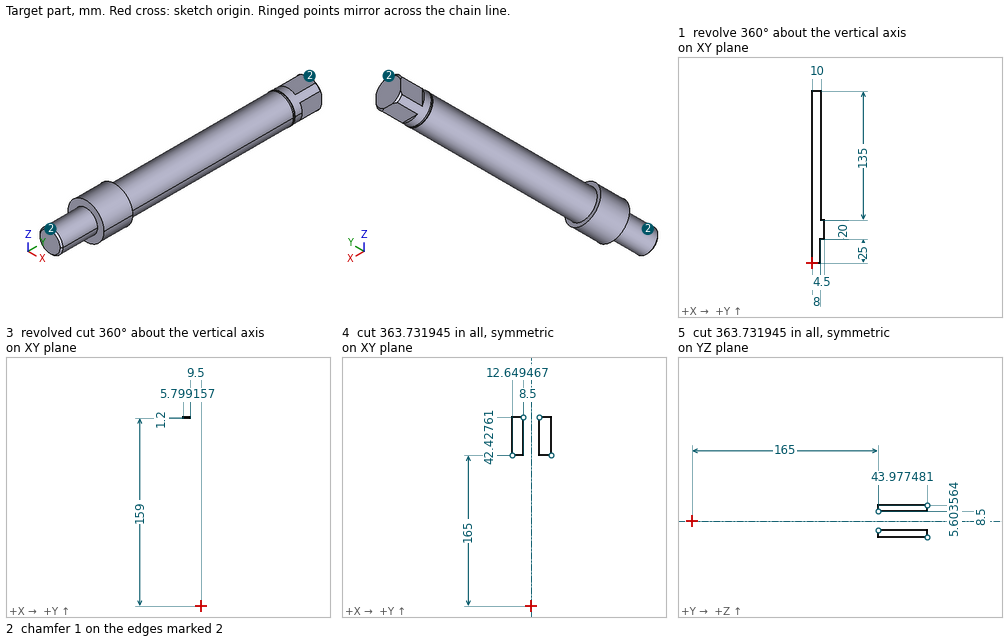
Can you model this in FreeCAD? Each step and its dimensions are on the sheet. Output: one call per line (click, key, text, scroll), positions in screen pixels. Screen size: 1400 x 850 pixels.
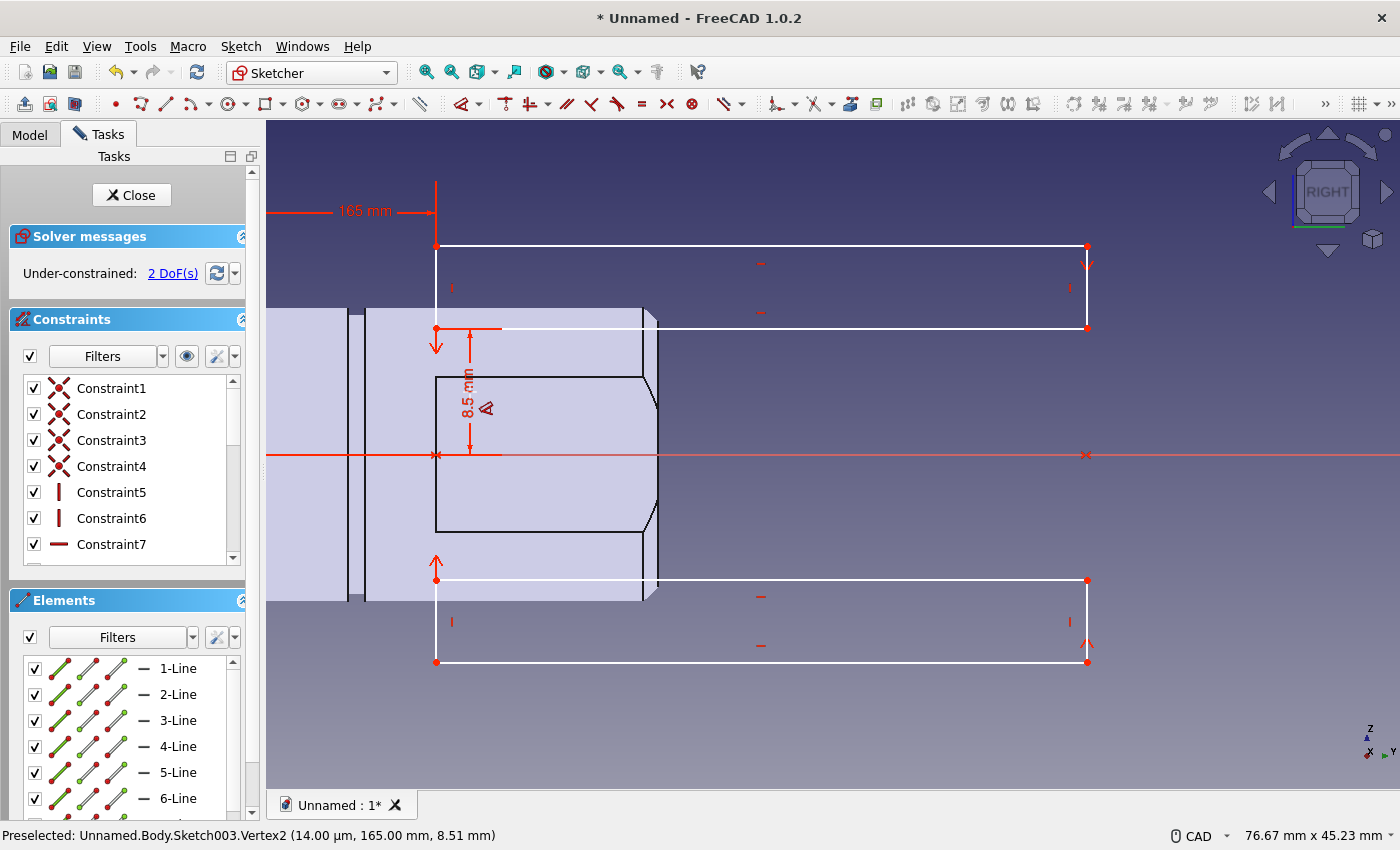
click(436, 271)
click(402, 288)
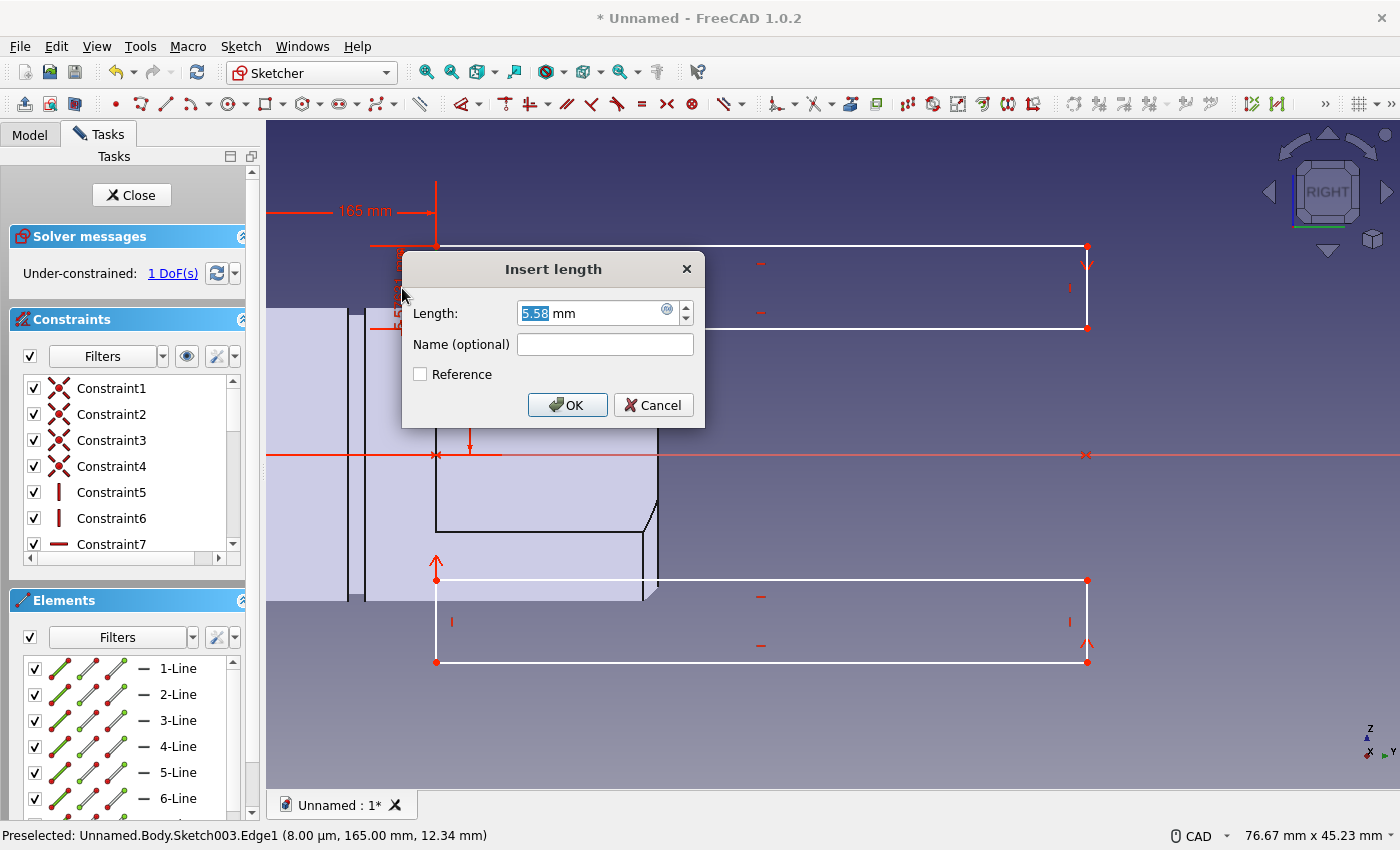
text(5.603564)
key(Return)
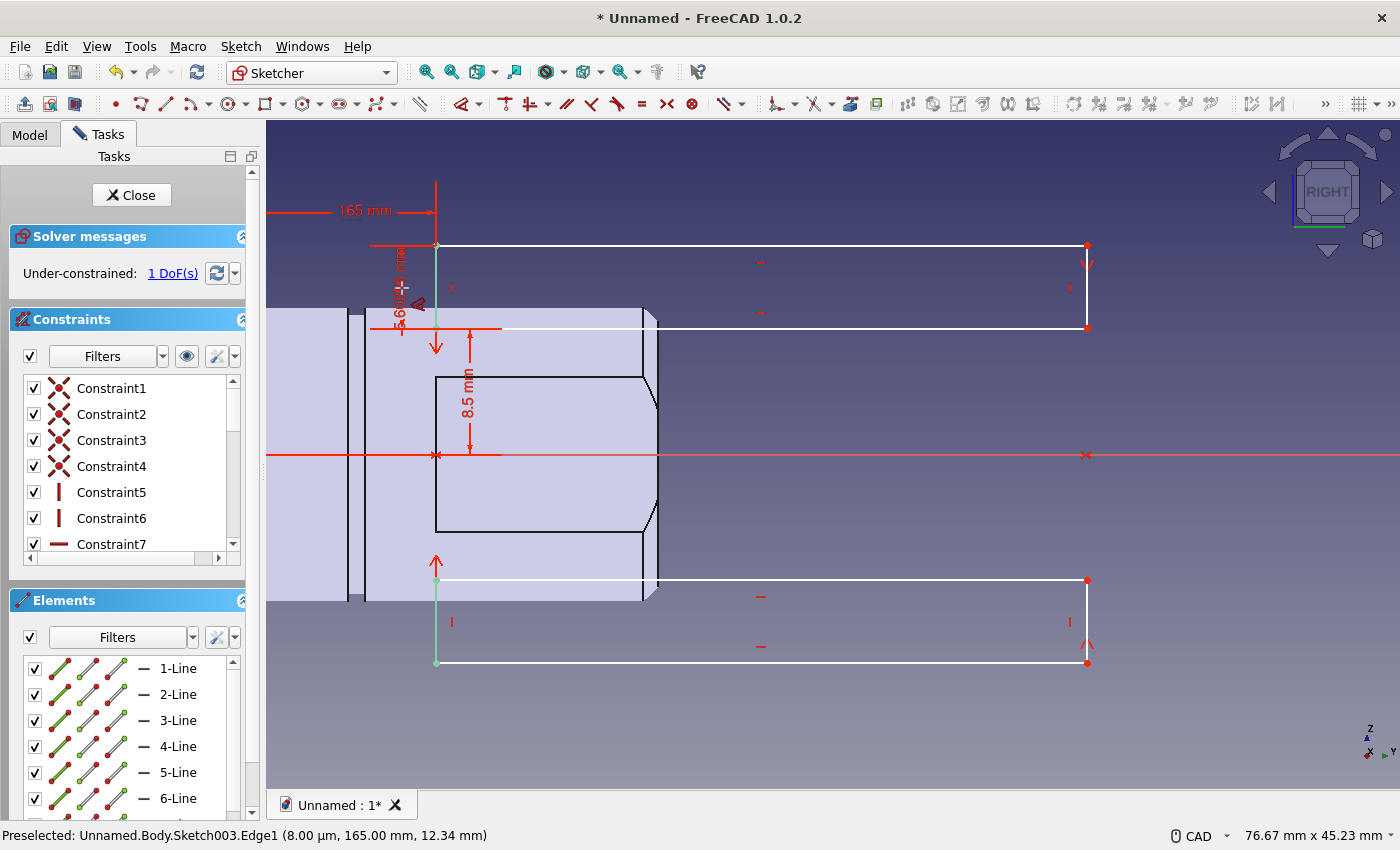
click(631, 329)
click(762, 295)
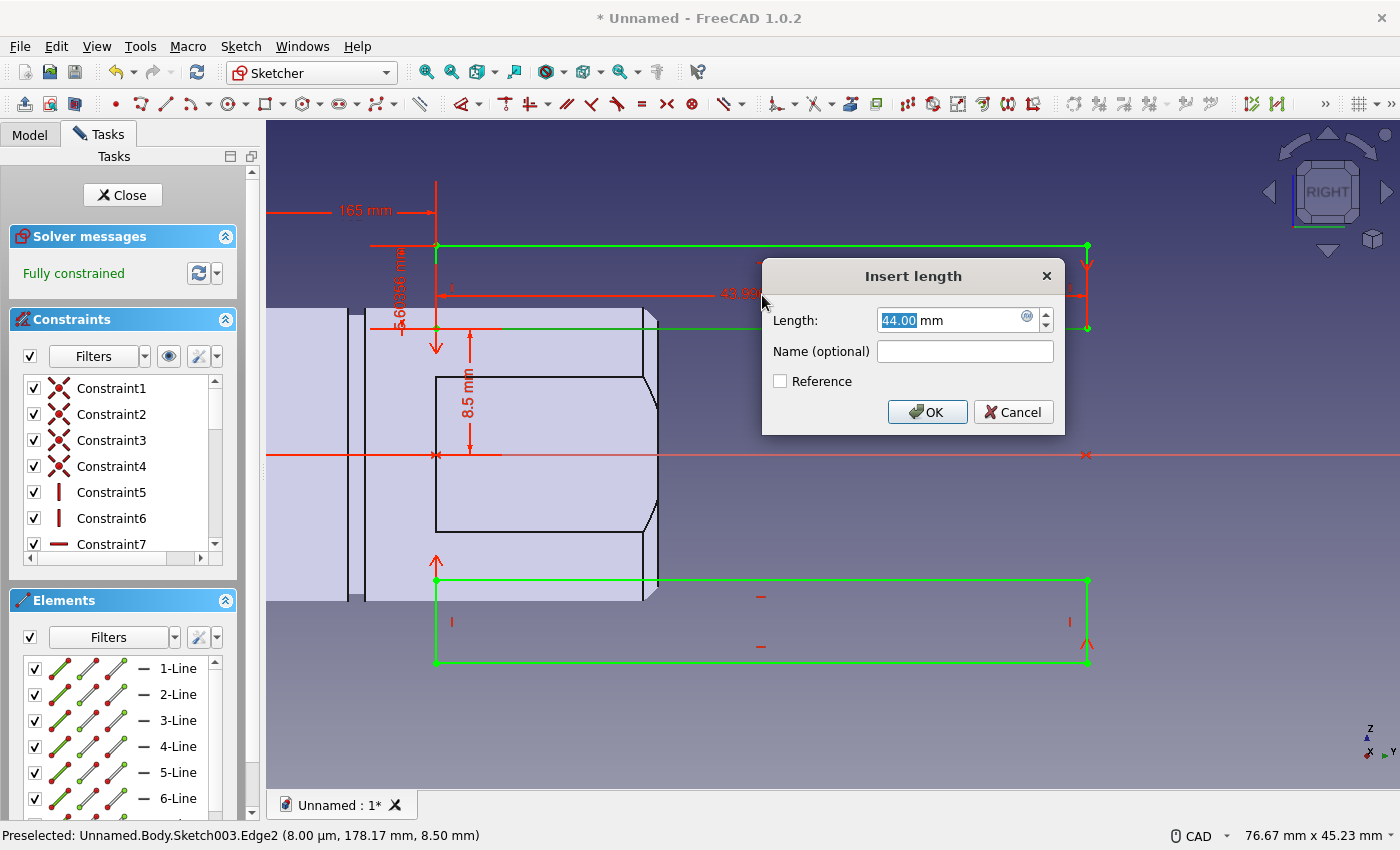
text(43.977481)
key(Return)
key(Escape)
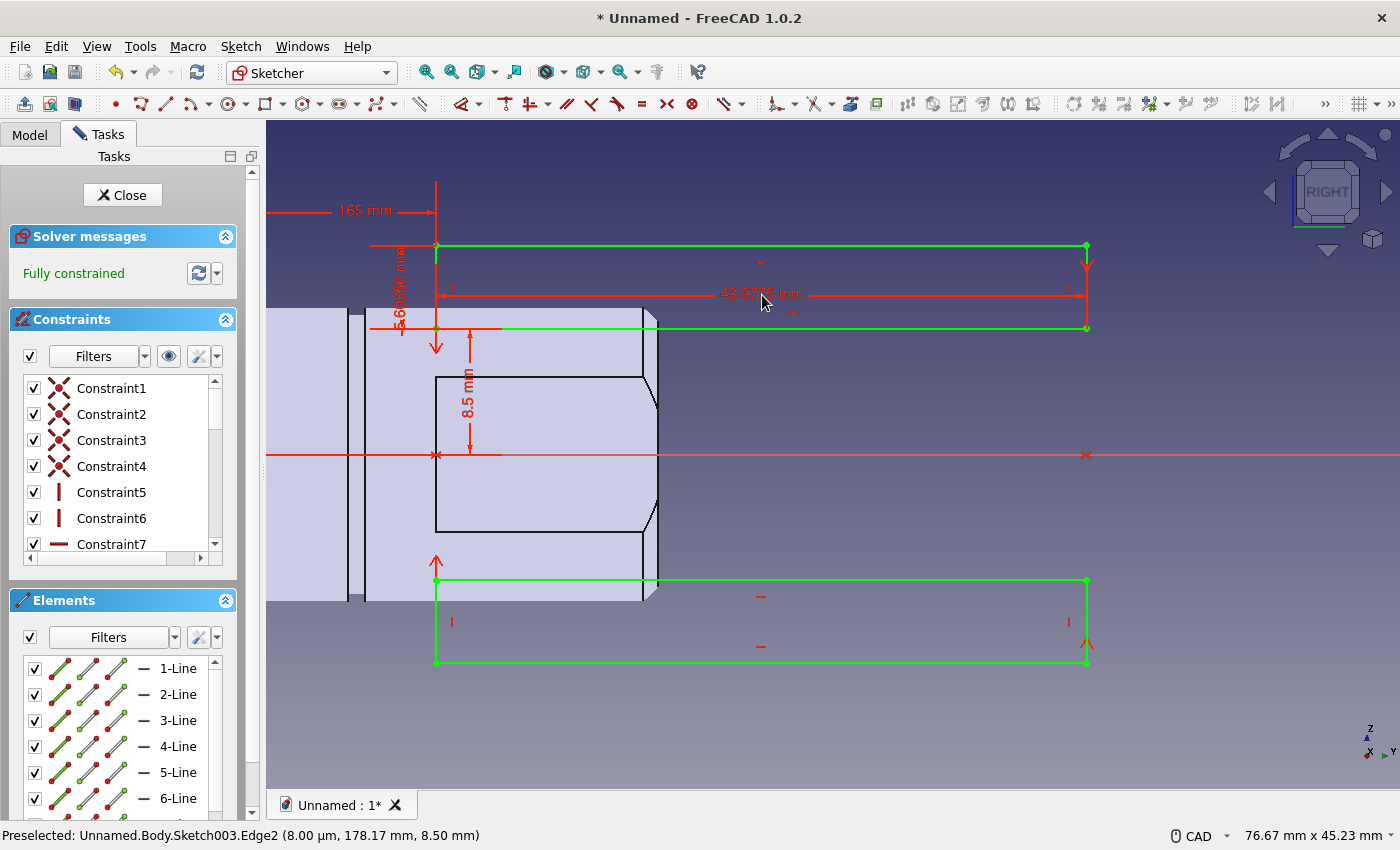
click(123, 195)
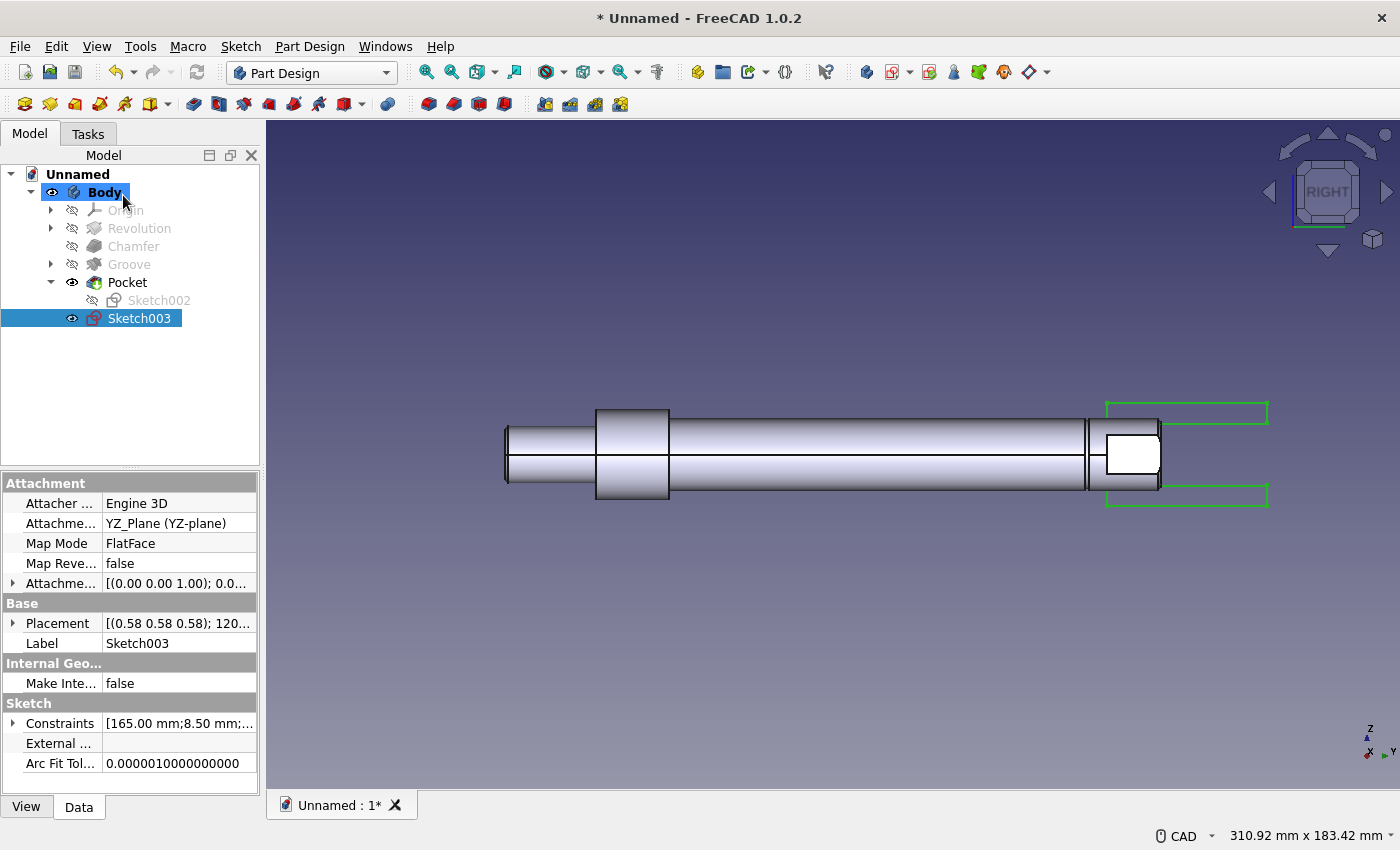
click(194, 104)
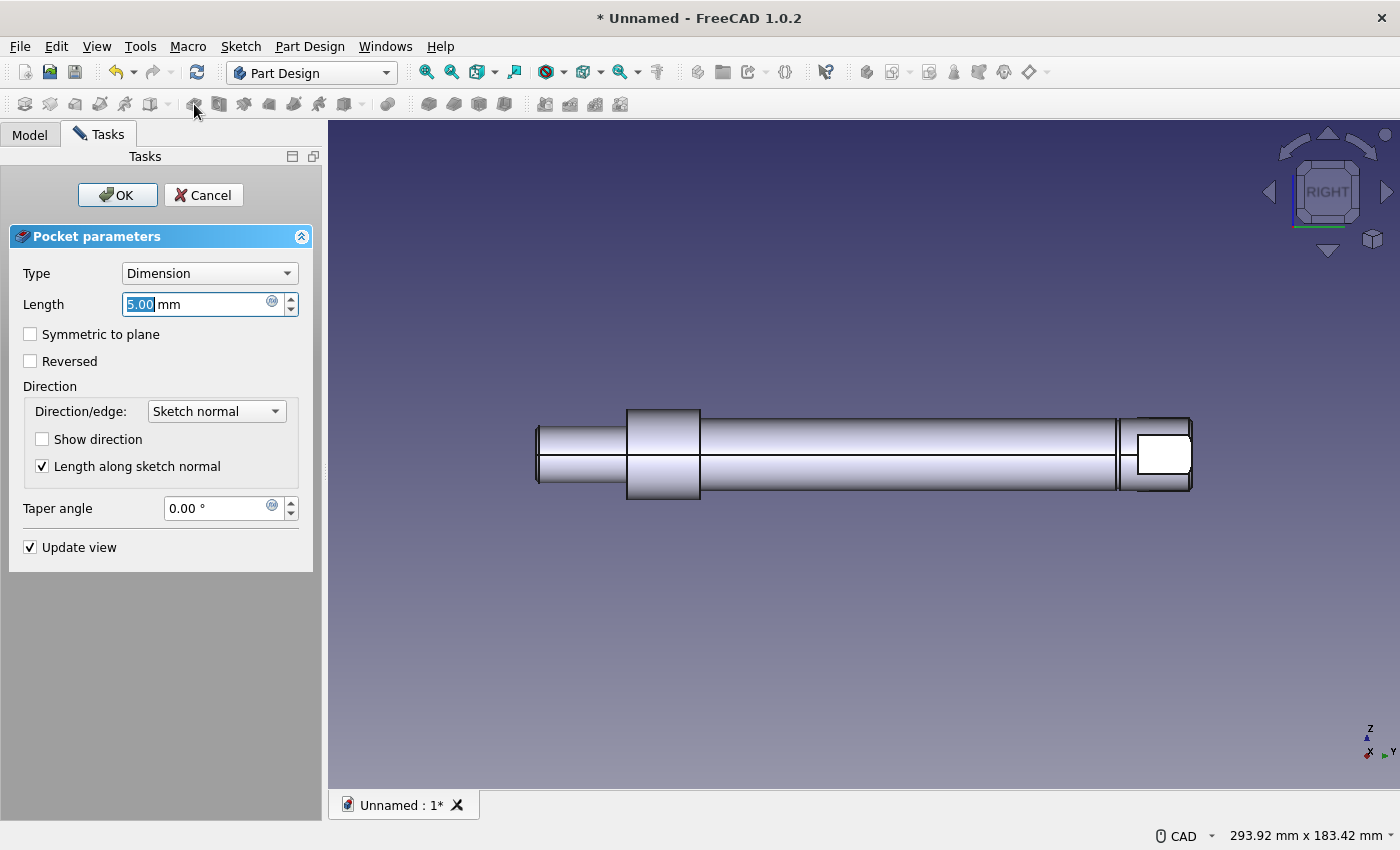
text(363.731945)
key(Tab)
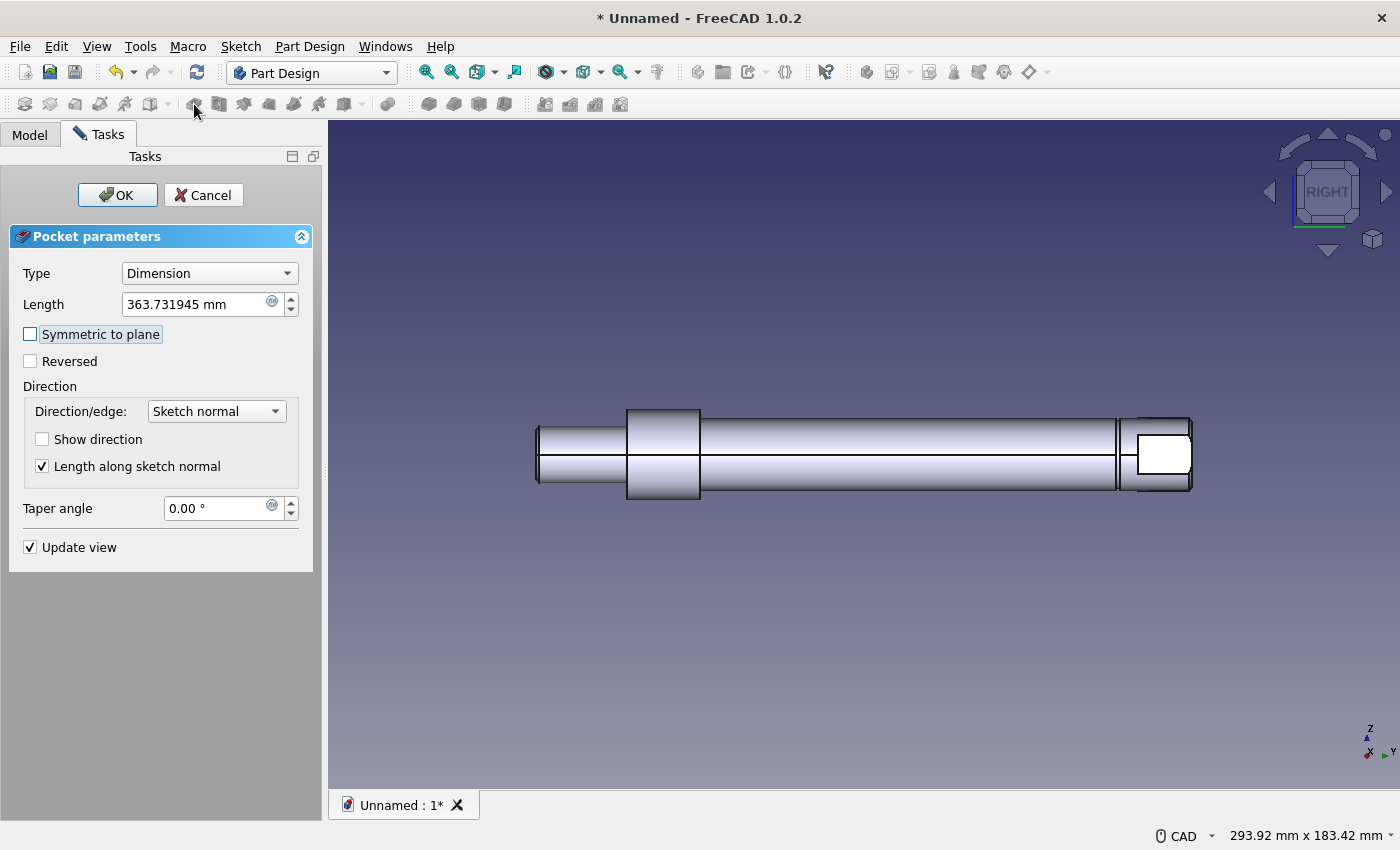
click(31, 334)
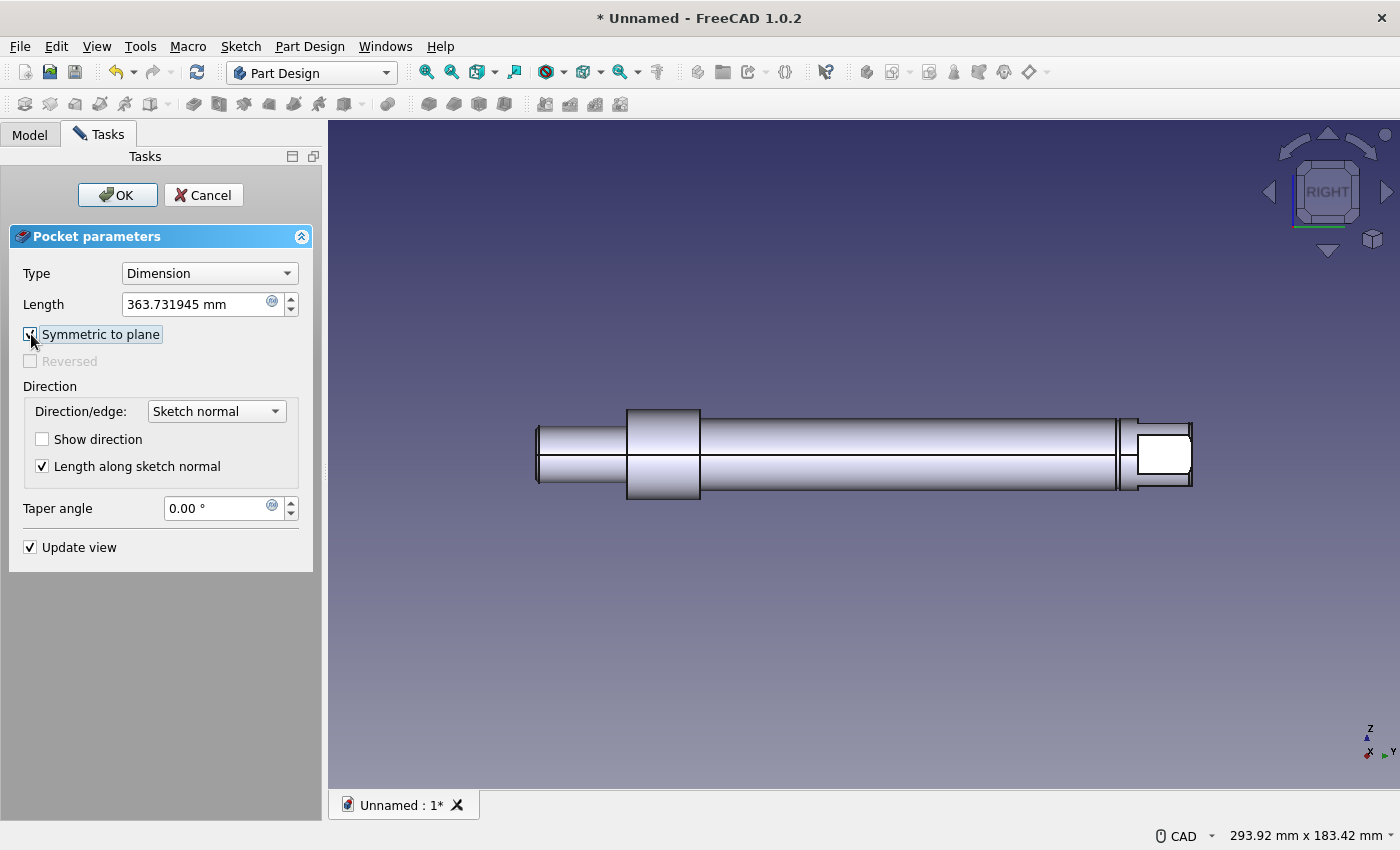
click(118, 195)